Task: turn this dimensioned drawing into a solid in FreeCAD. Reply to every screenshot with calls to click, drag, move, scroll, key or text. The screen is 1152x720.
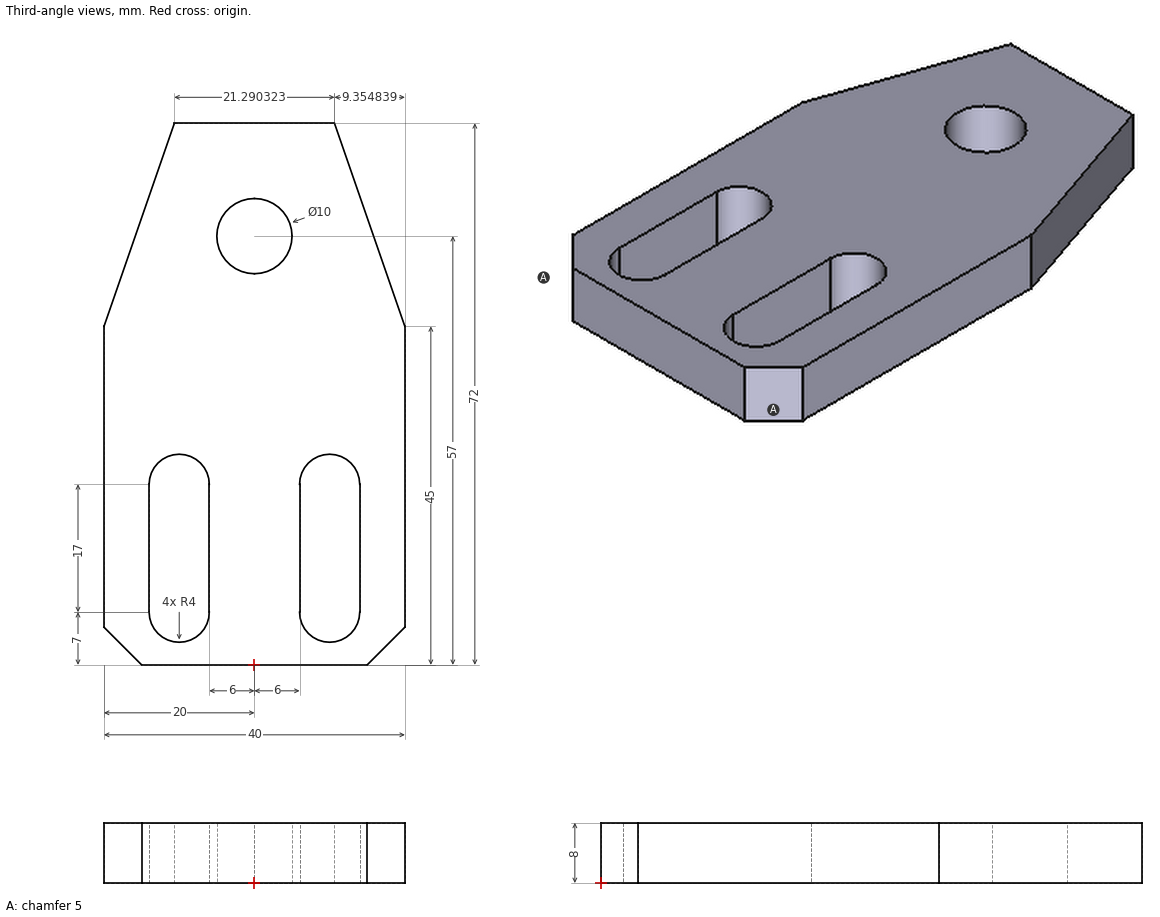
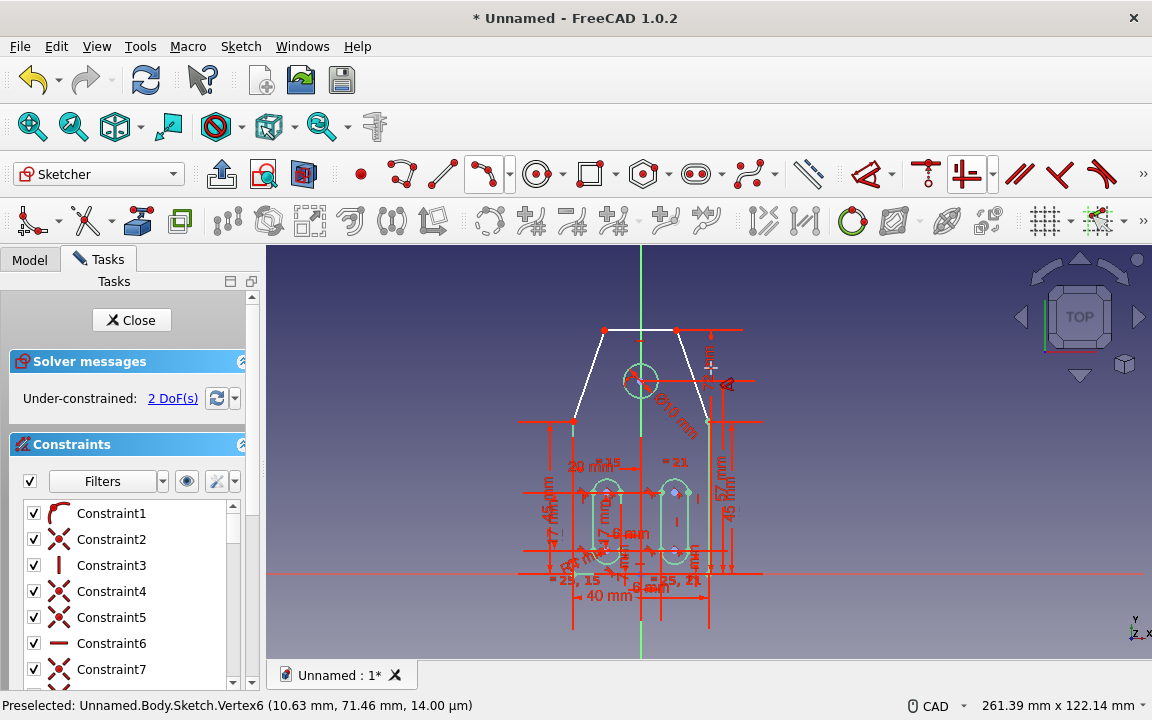
click(655, 330)
click(624, 296)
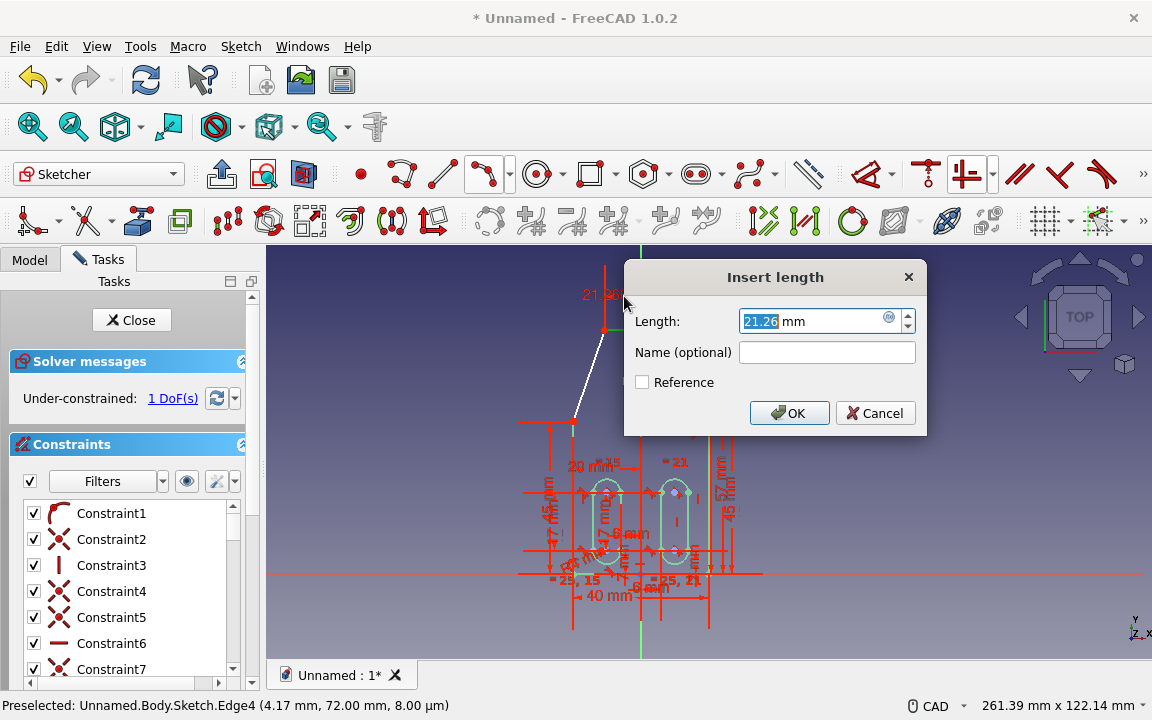
text(21.290323)
key(Return)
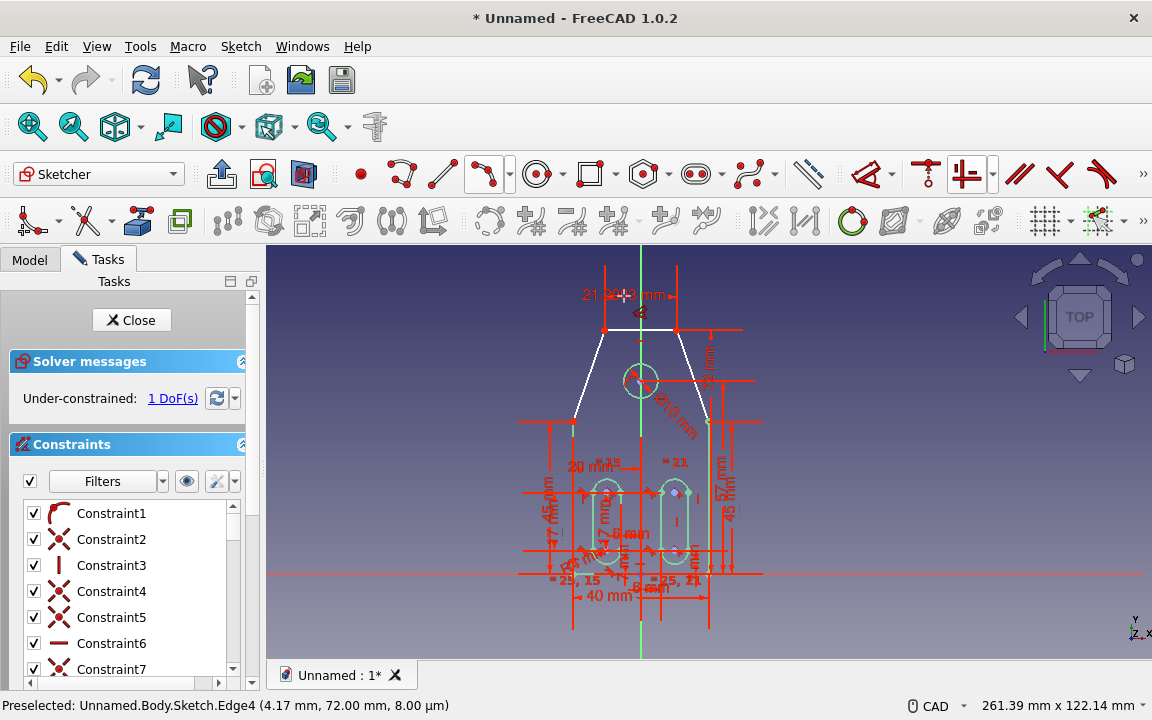
scroll(699, 394, up, 2)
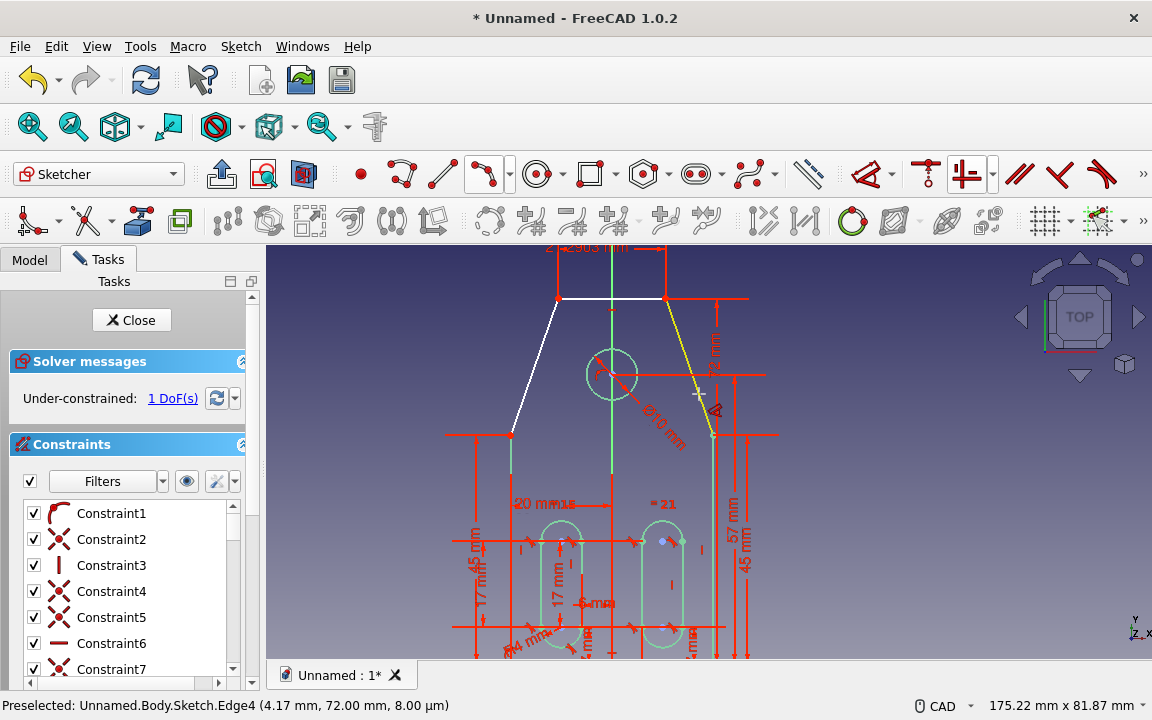
click(699, 394)
click(690, 469)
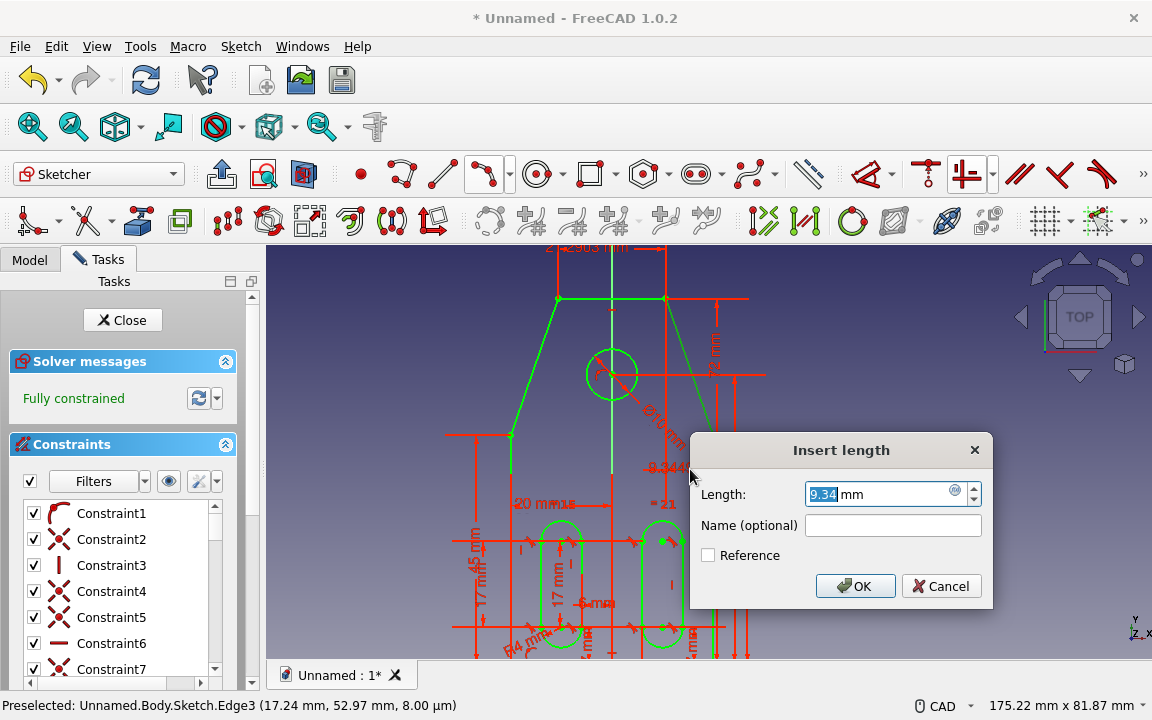
text(9.354839)
key(Return)
key(Escape)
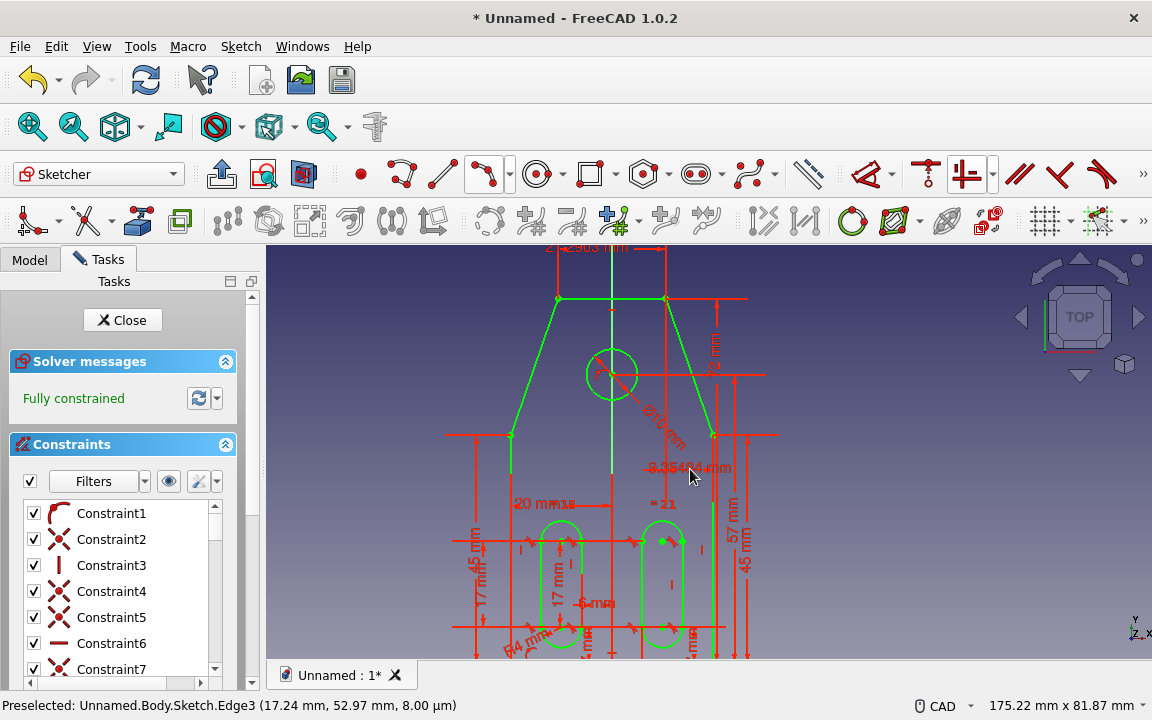
click(123, 320)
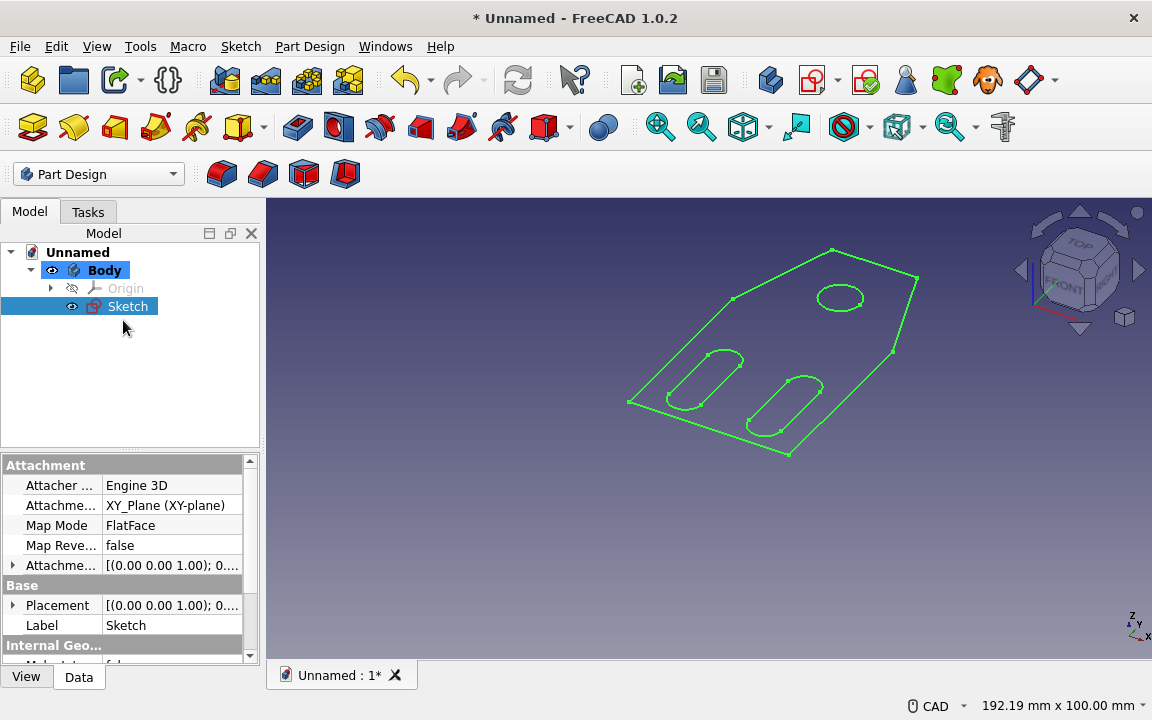
click(33, 128)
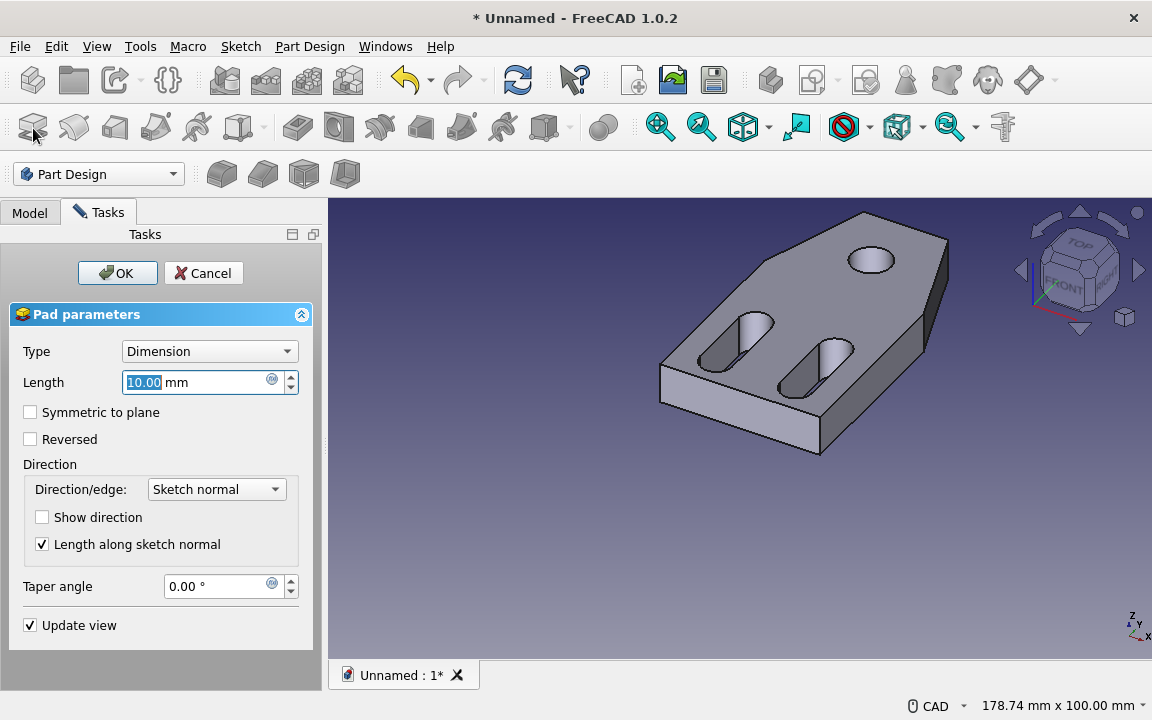
text(8)
key(Tab)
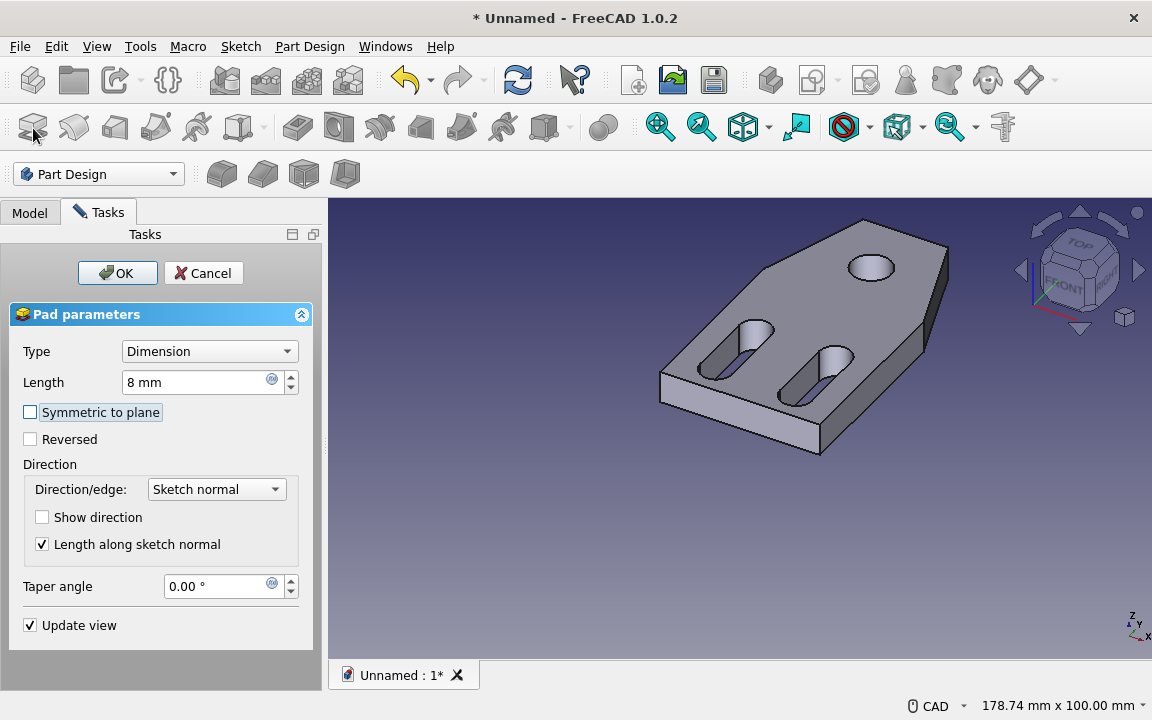
click(118, 273)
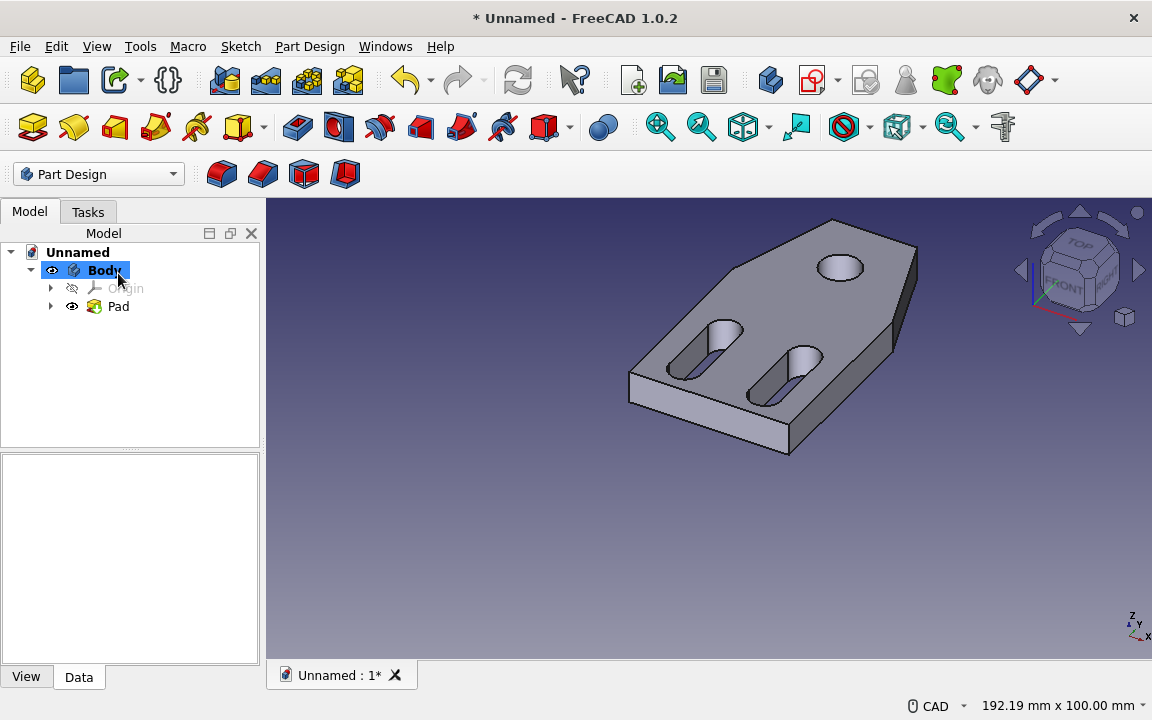
click(789, 439)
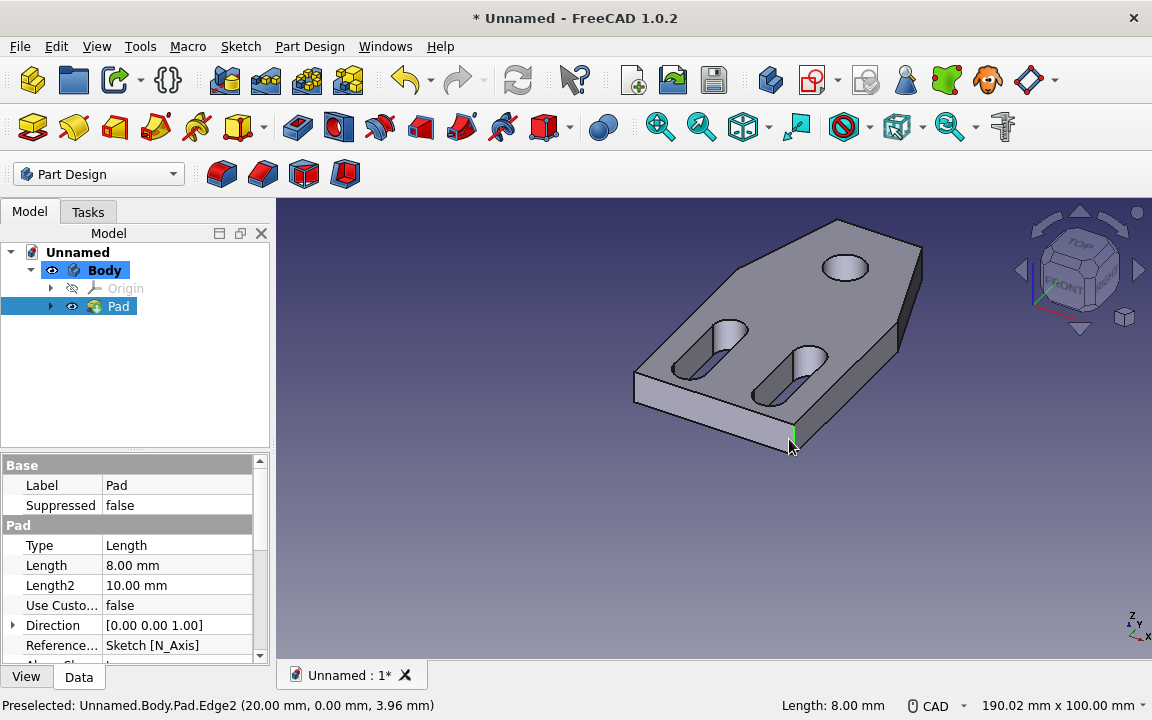
key(0)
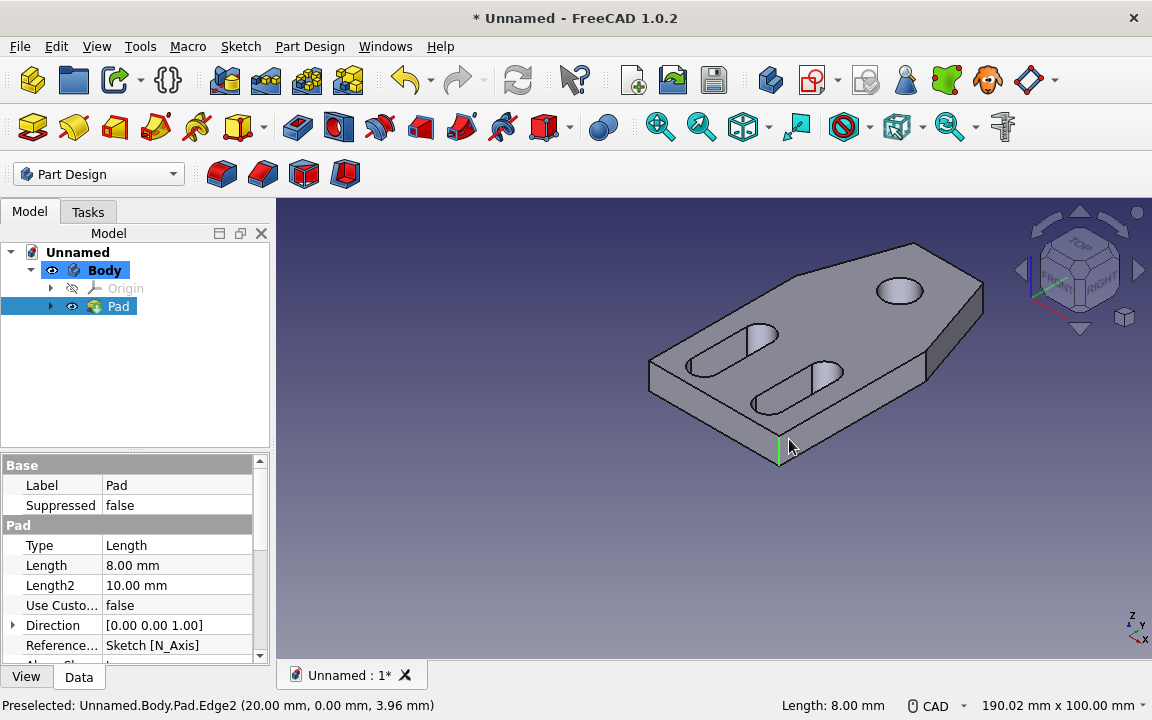
key(2)